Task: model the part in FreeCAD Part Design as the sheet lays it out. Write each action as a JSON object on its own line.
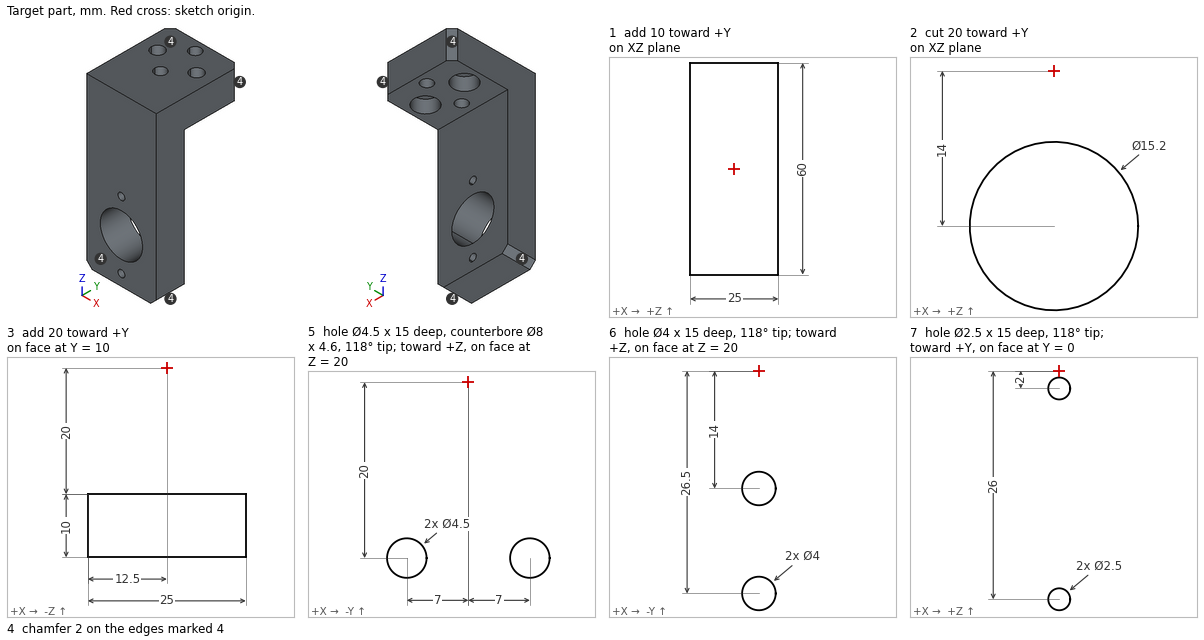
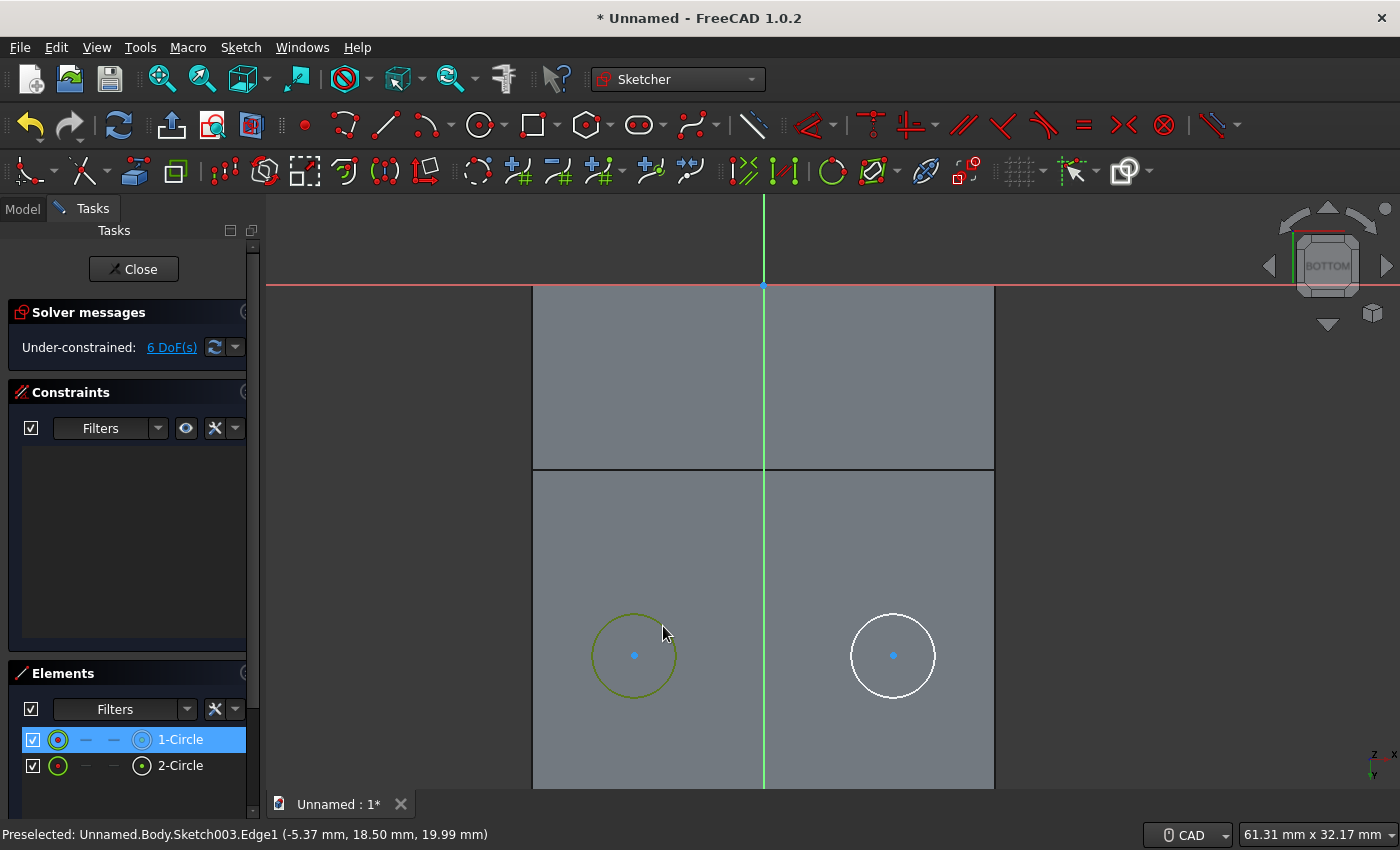
{"action": "left_click", "coordinate": [922, 626]}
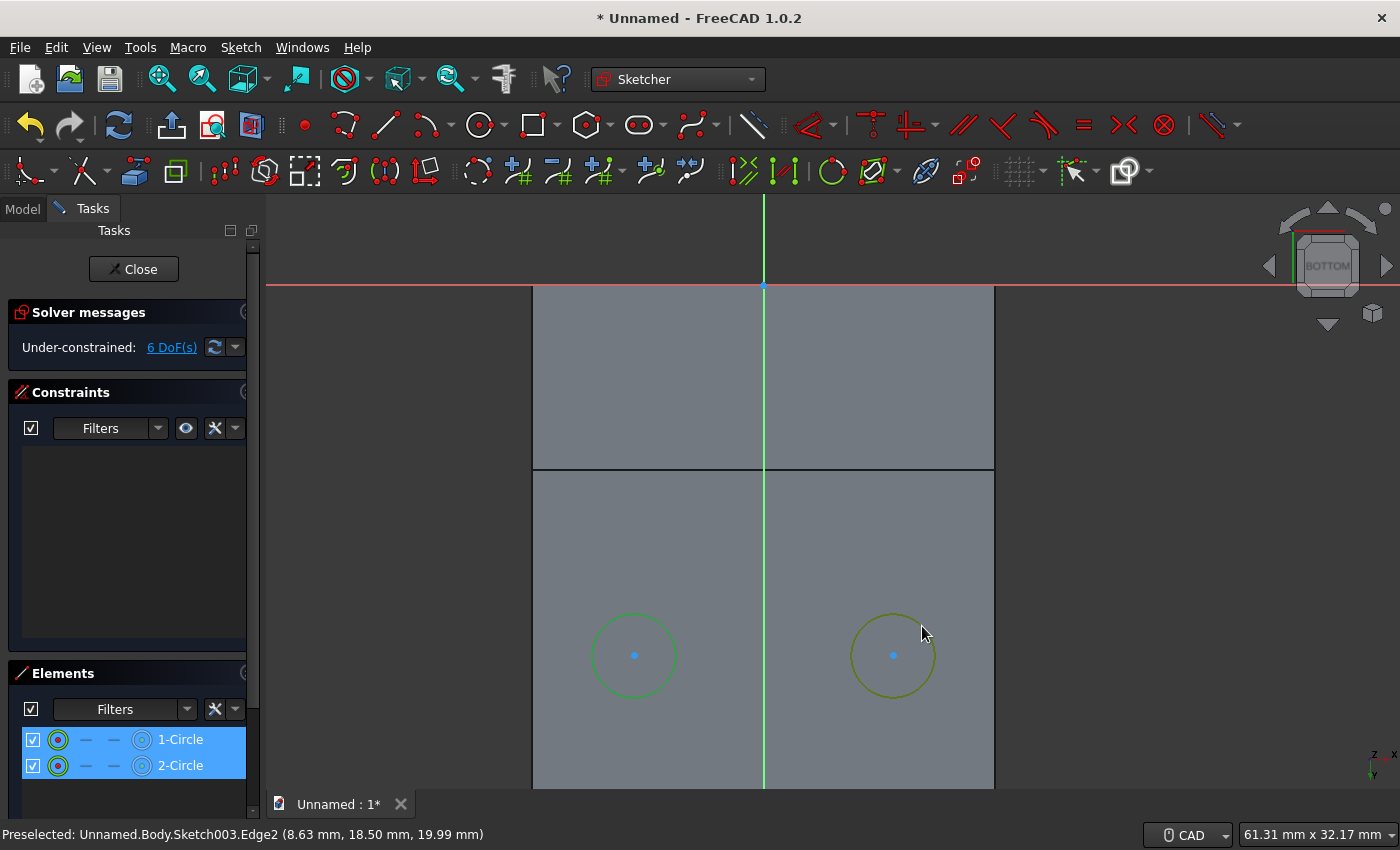
{"action": "key", "text": "e"}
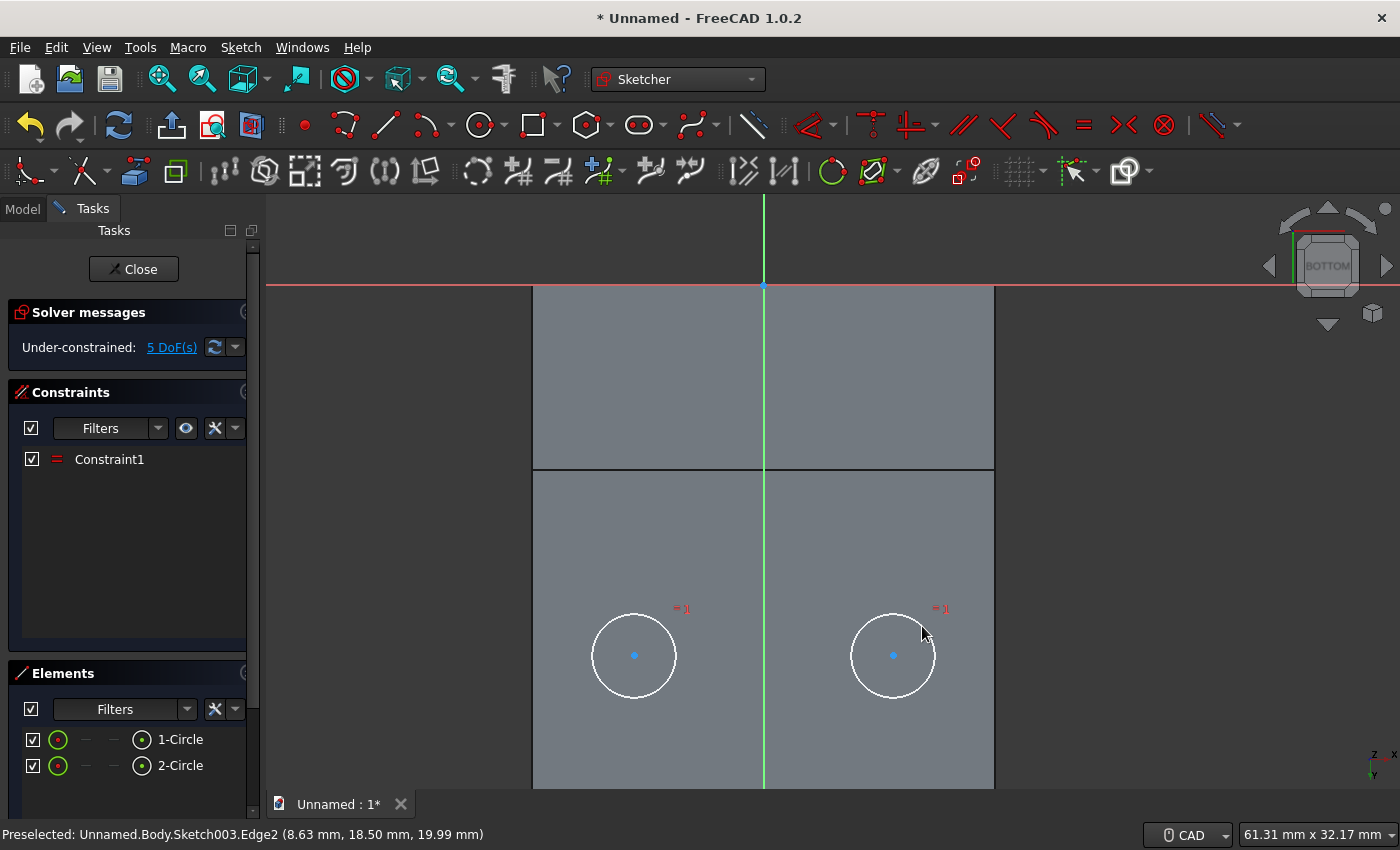
{"action": "left_click", "coordinate": [634, 656]}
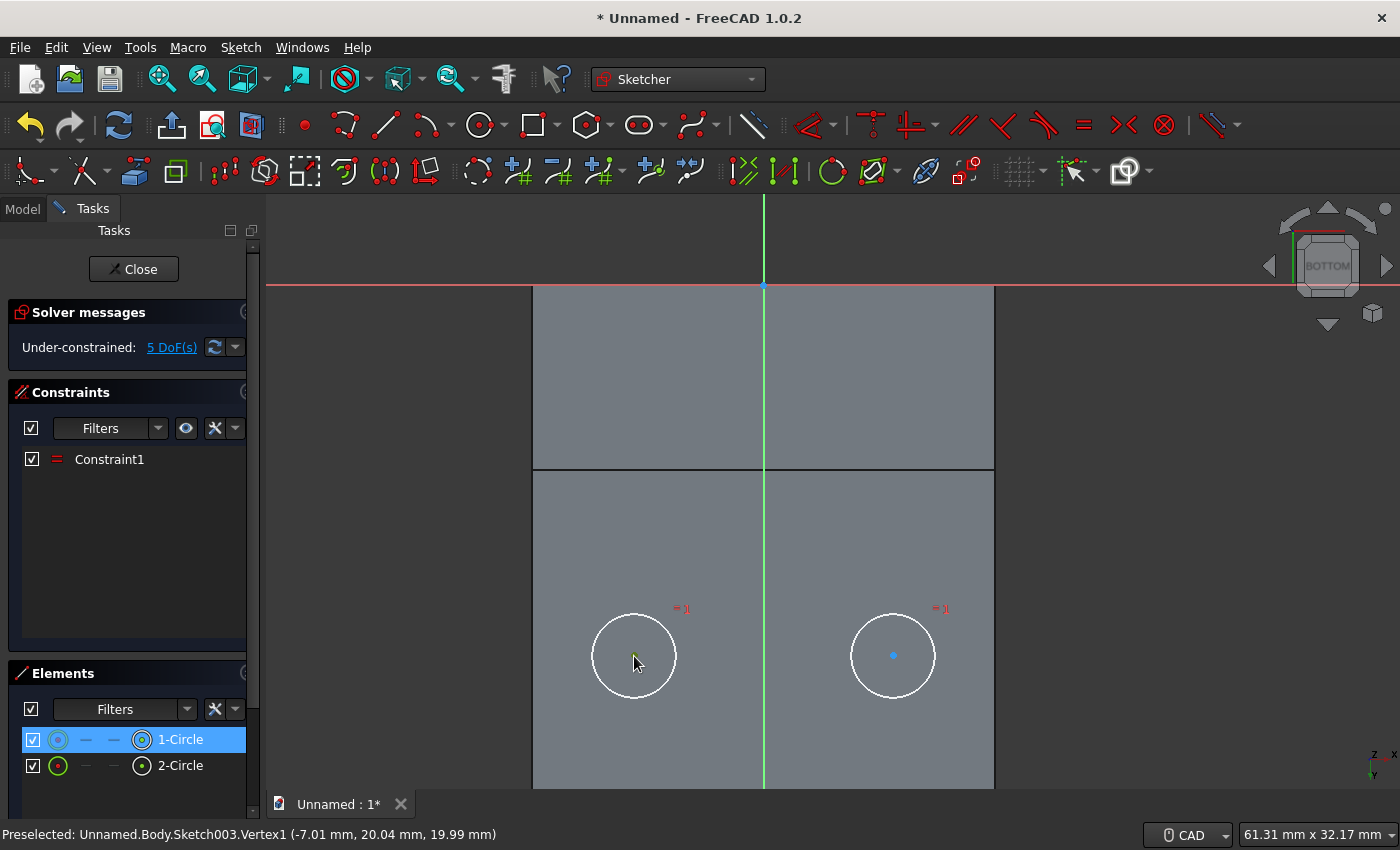
{"action": "left_click", "coordinate": [893, 656]}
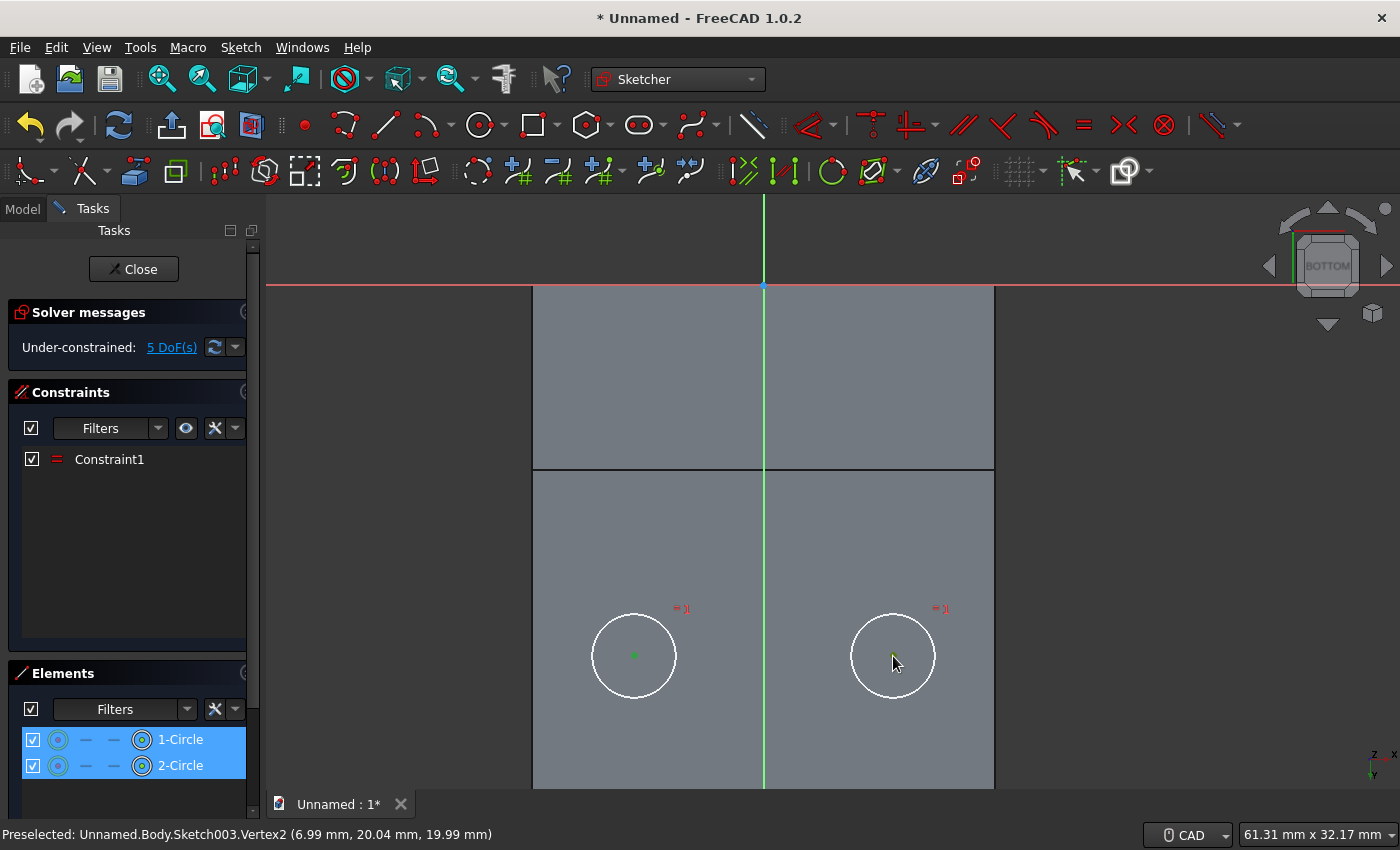
{"action": "key", "text": "h"}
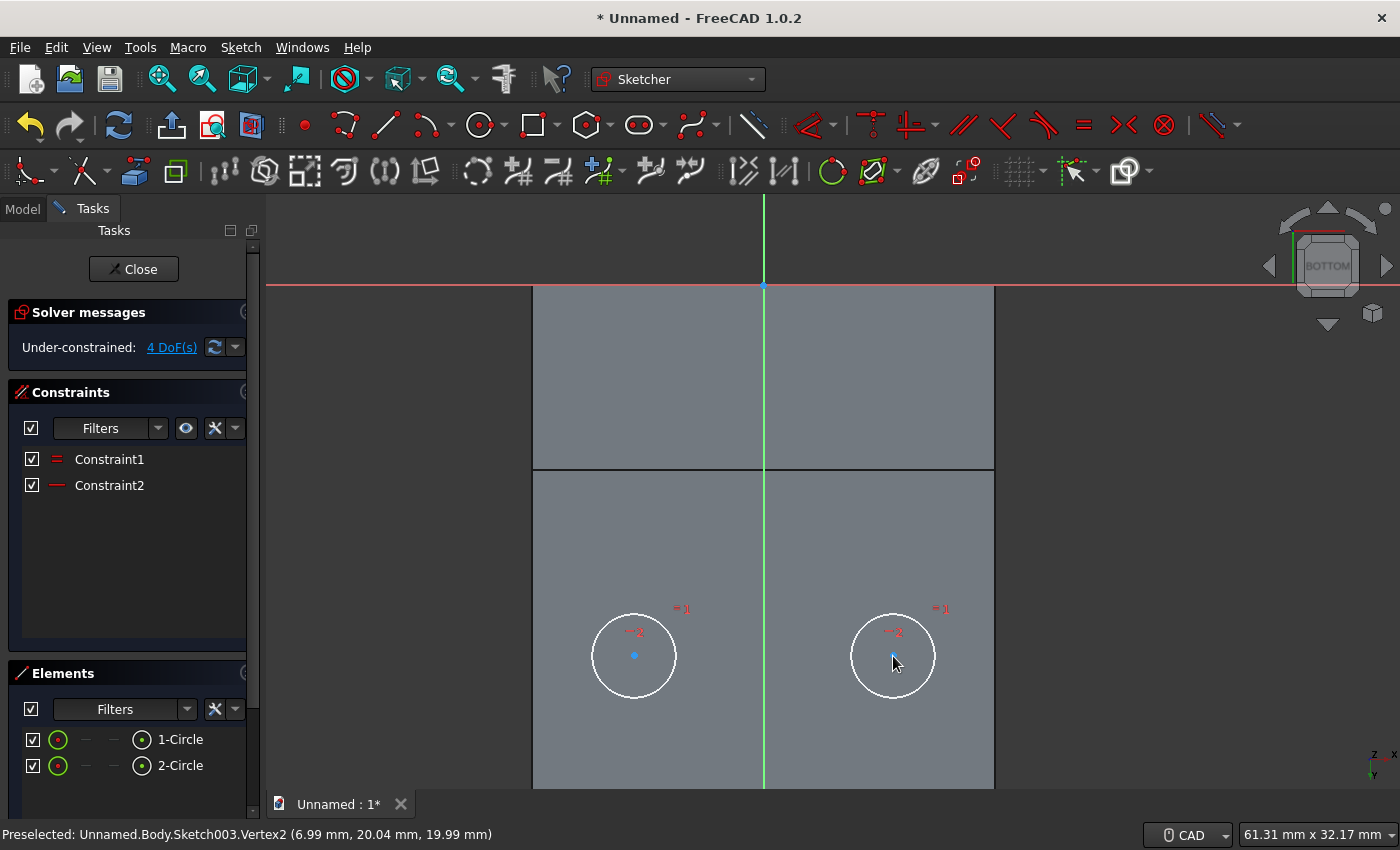
{"action": "key", "text": "d"}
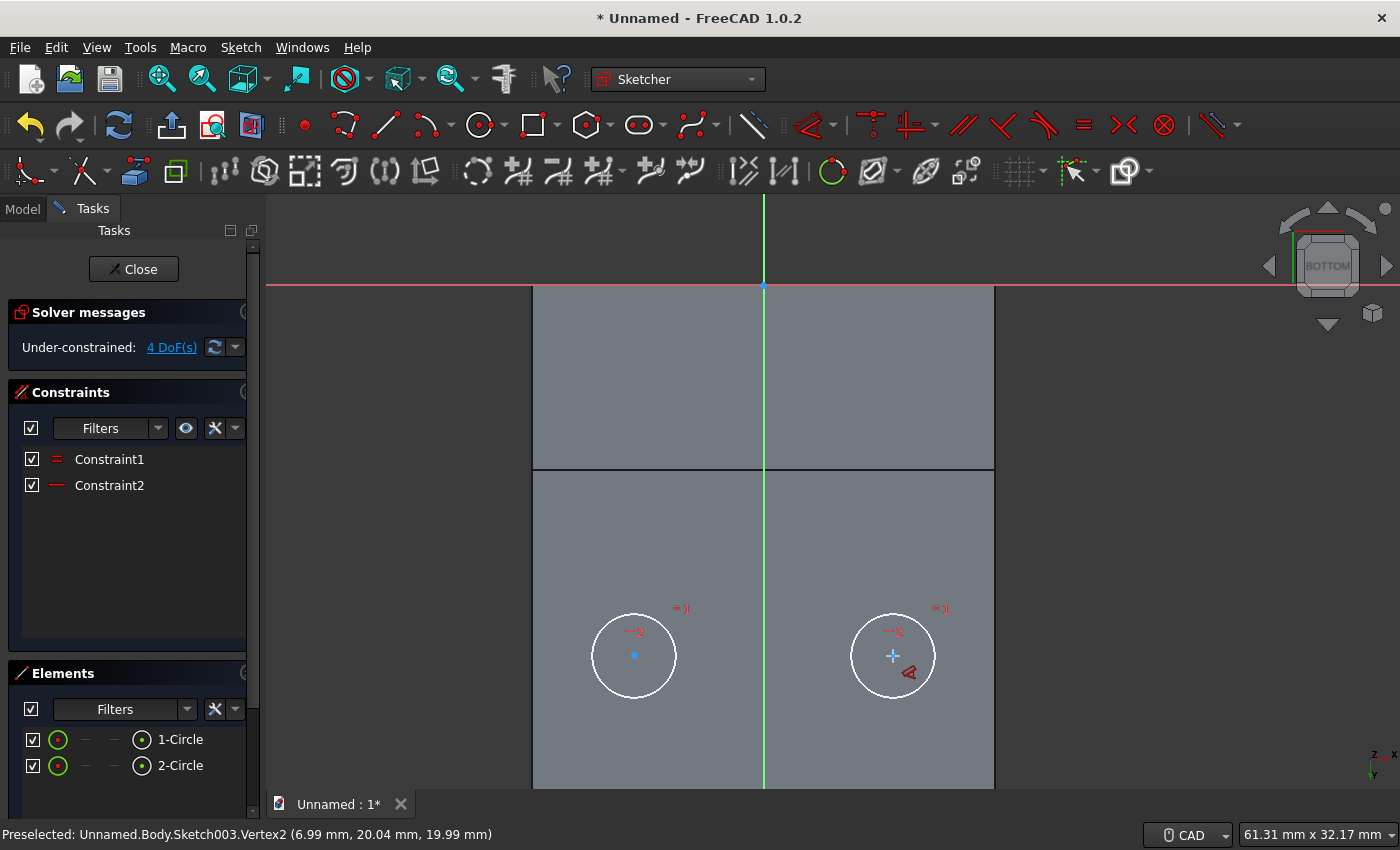
{"action": "left_click", "coordinate": [663, 626]}
{"action": "left_click", "coordinate": [685, 603]}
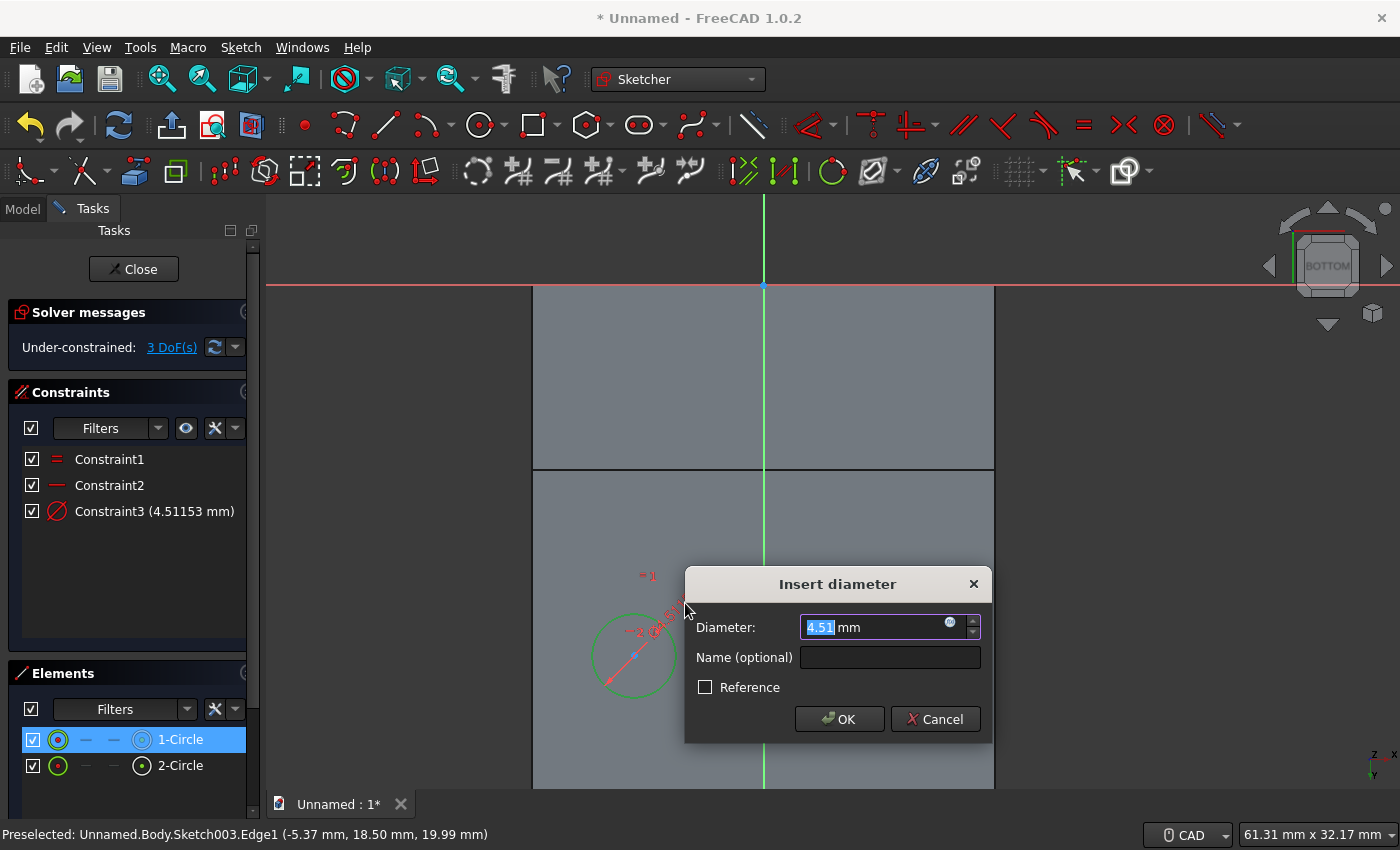
{"action": "type", "text": "4.5"}
{"action": "key", "text": "Return"}